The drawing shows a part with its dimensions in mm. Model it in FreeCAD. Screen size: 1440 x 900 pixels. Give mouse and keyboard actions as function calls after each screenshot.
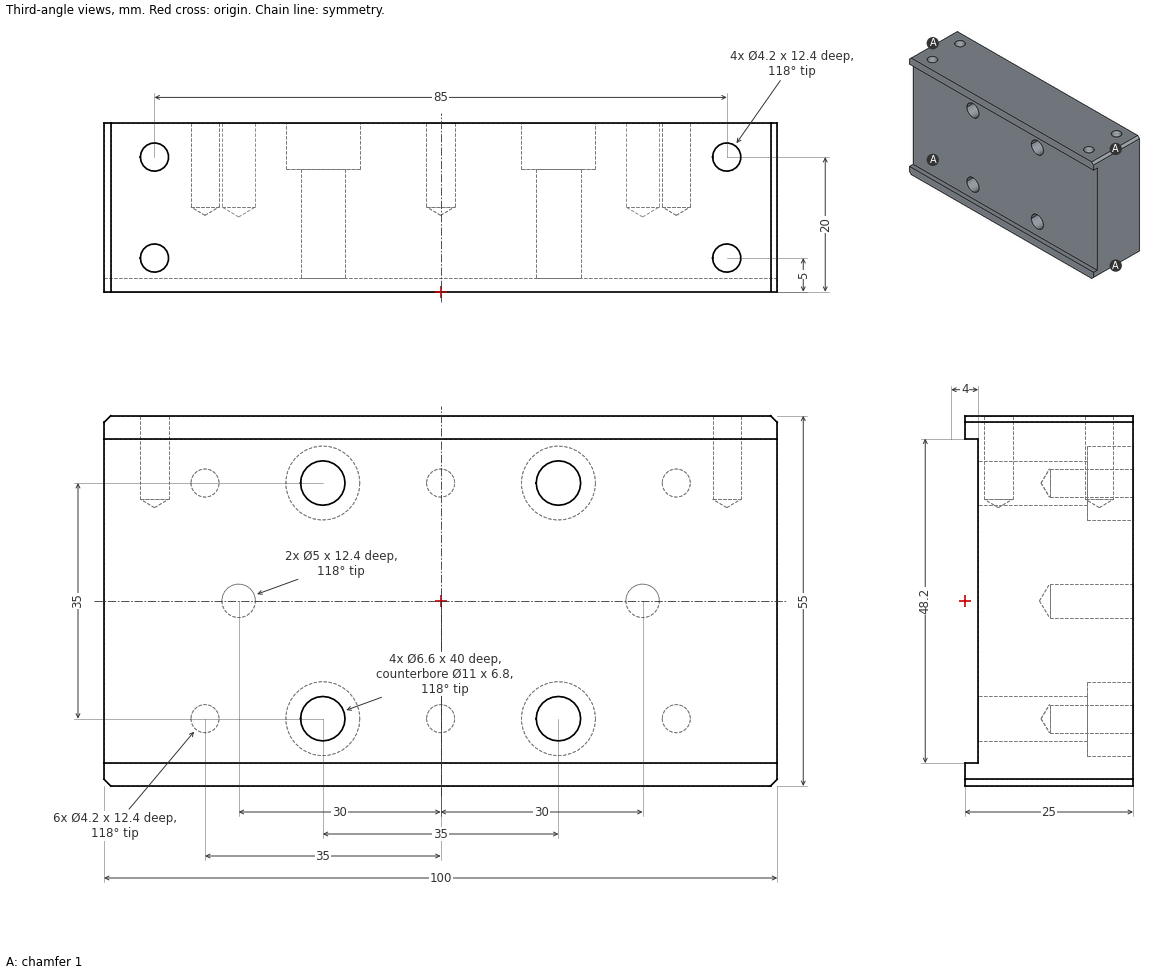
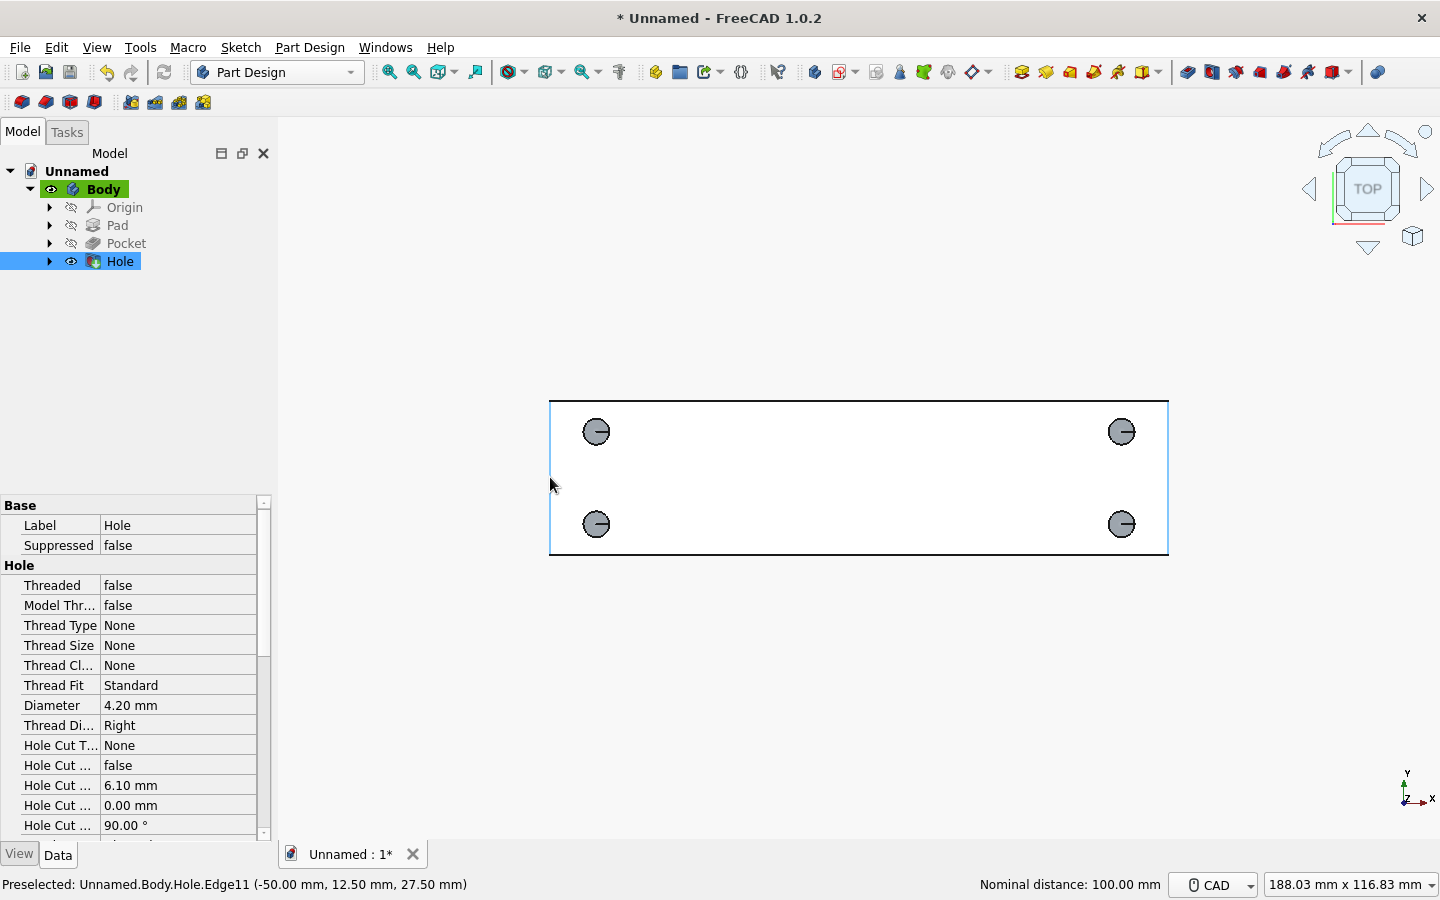
key(1)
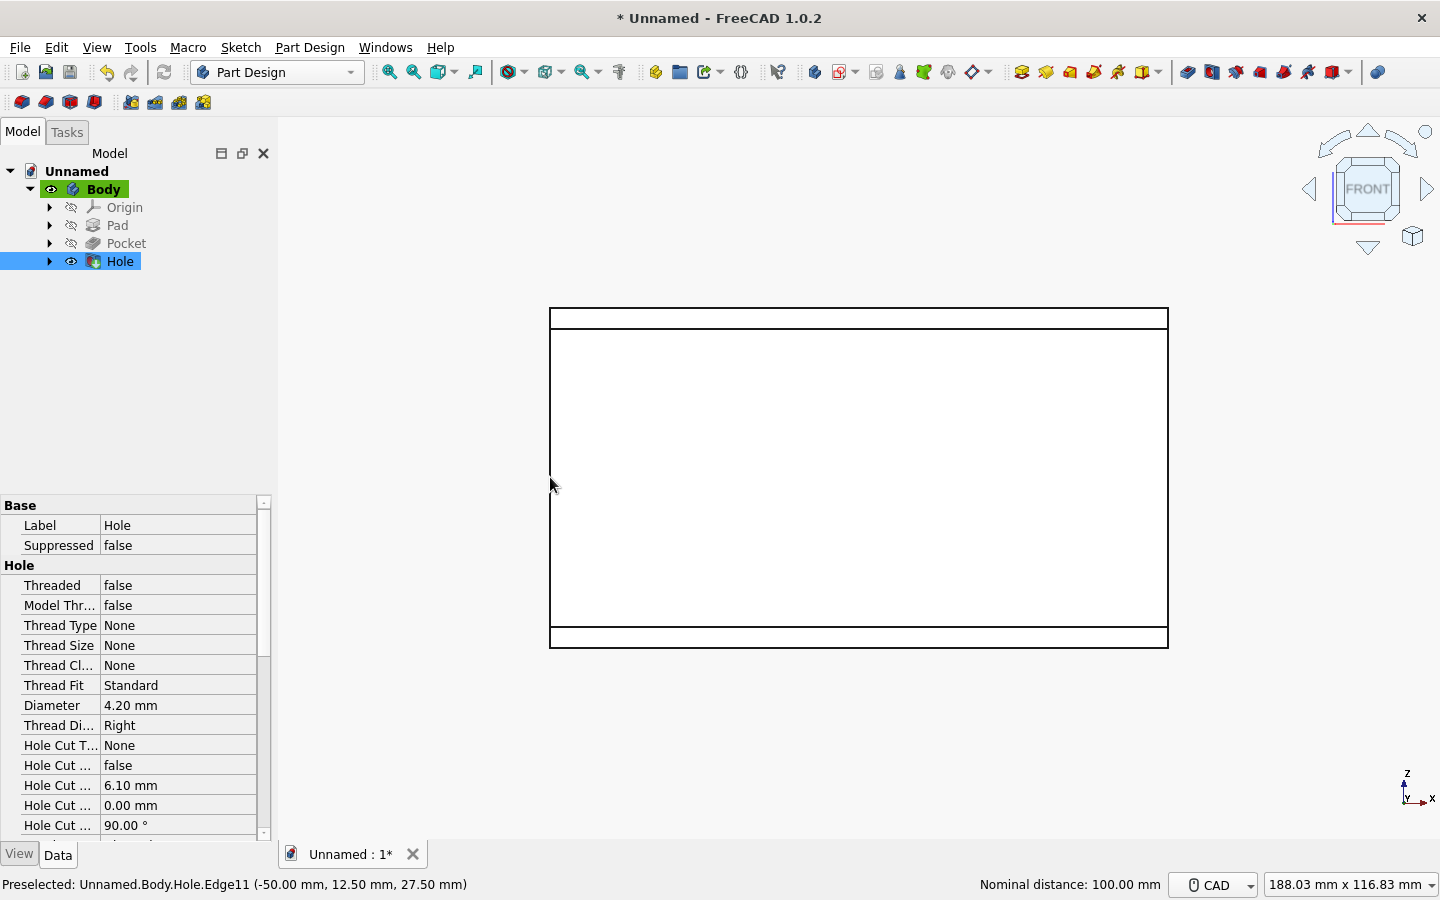
key(3)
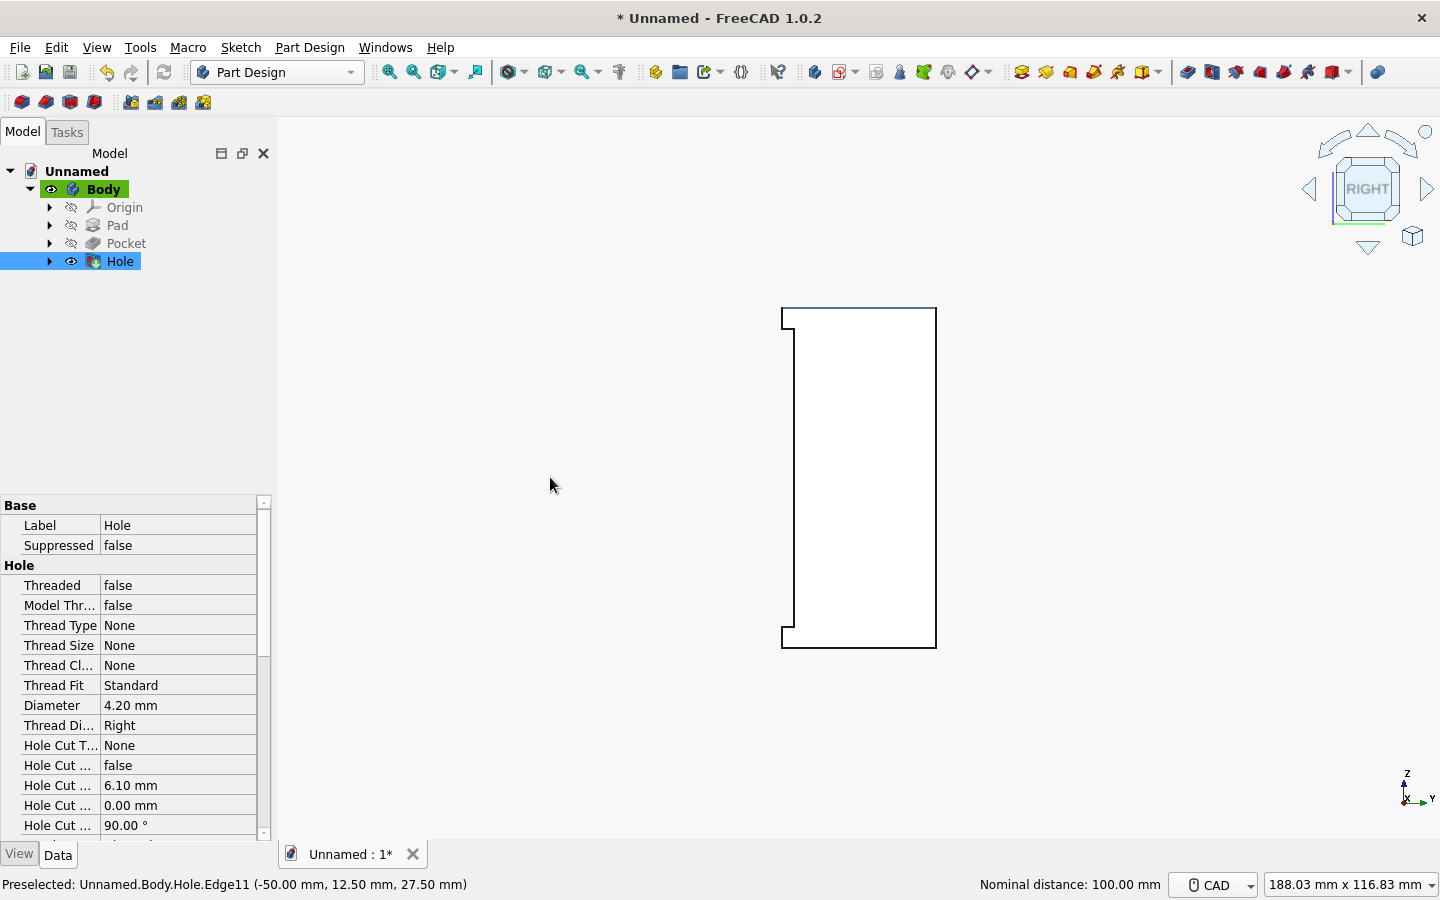
click(859, 647, ctrl)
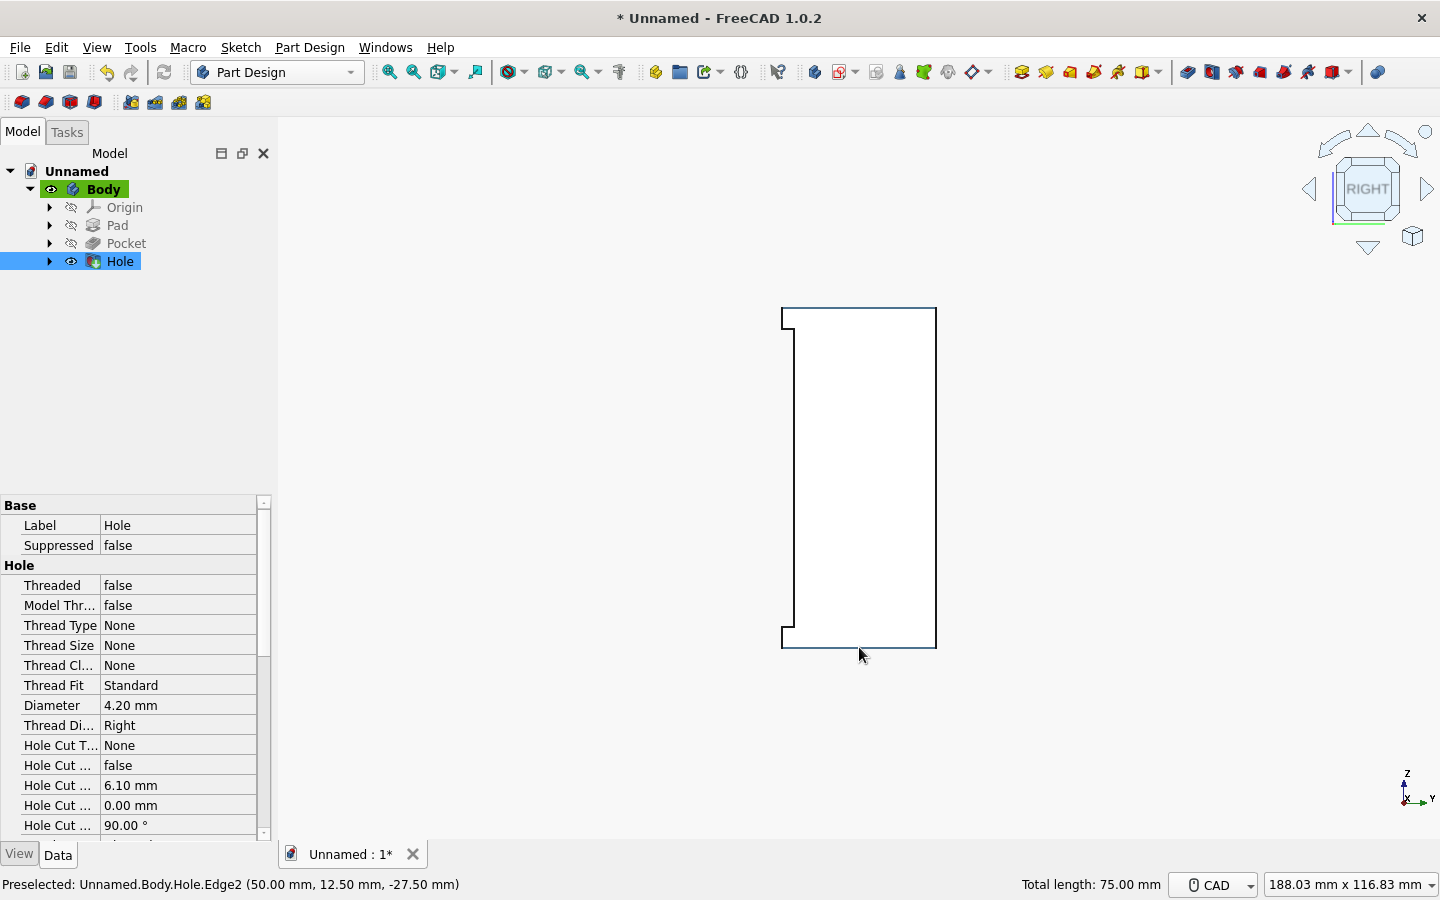
key(5)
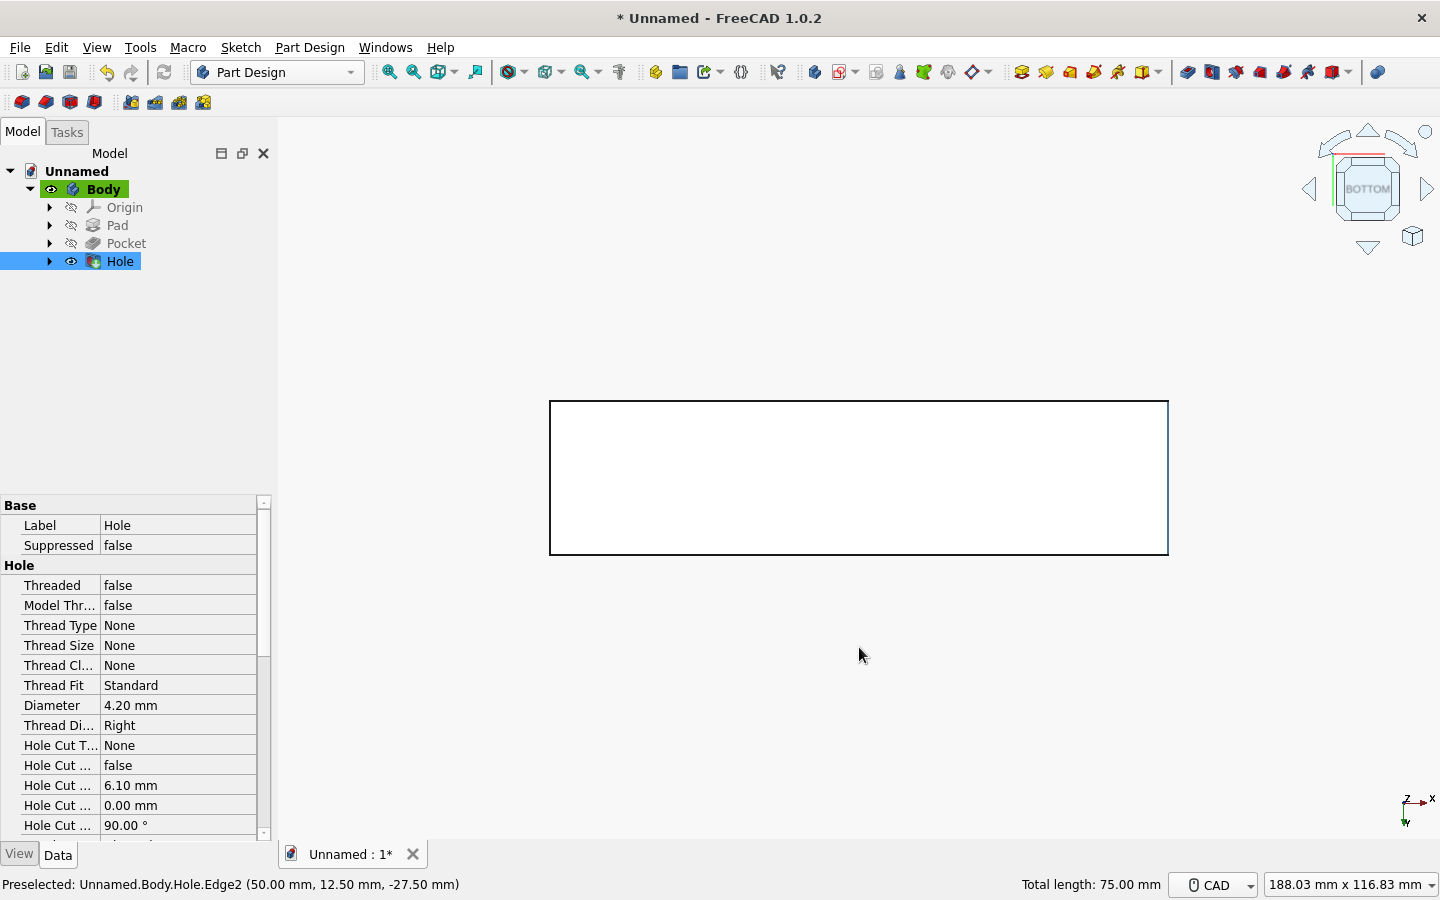
click(550, 477, ctrl)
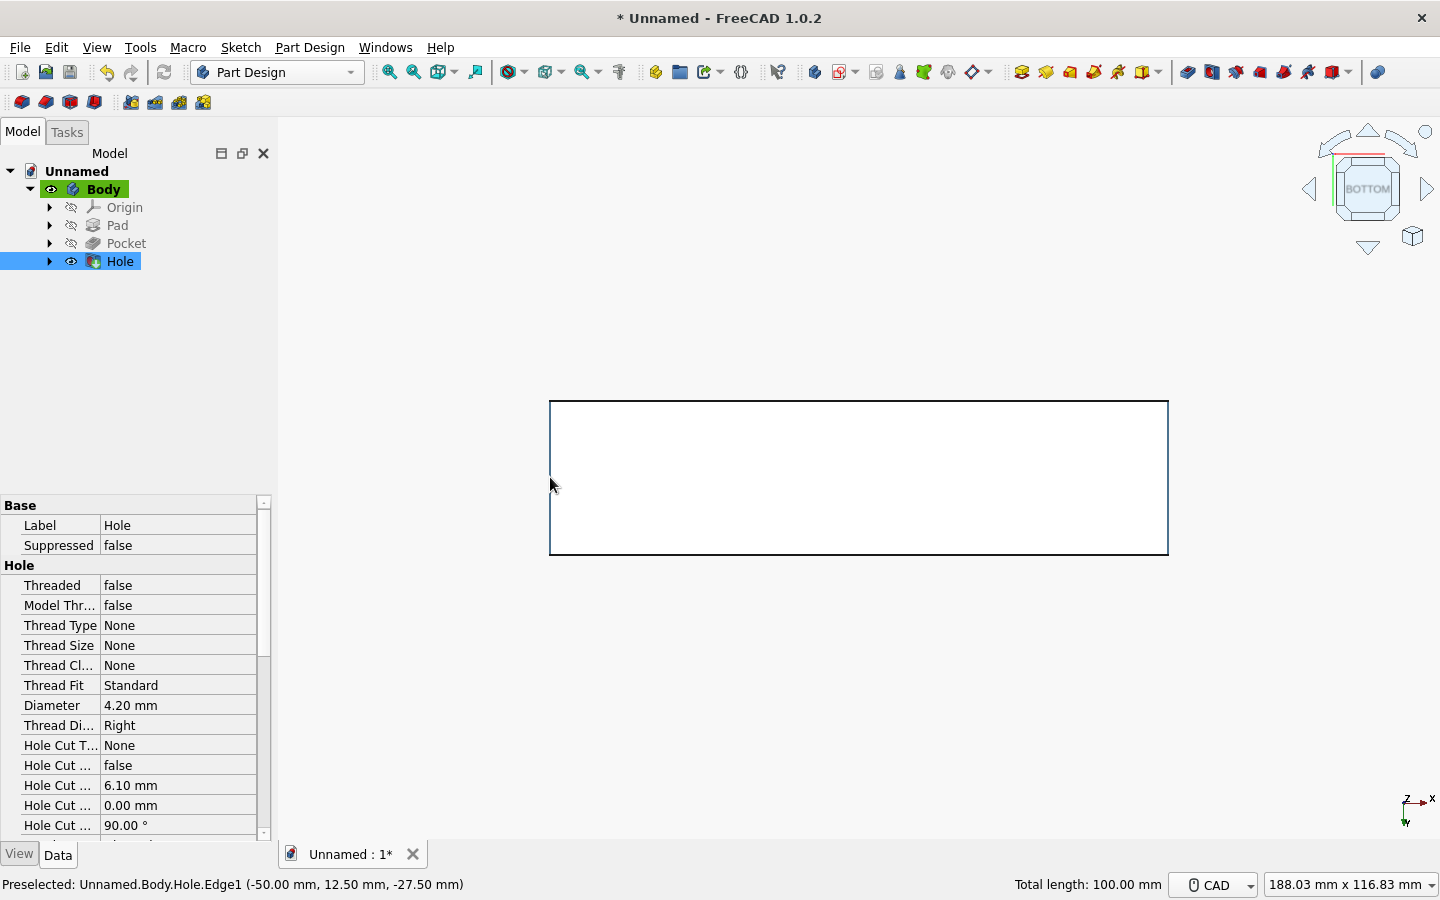
click(46, 102)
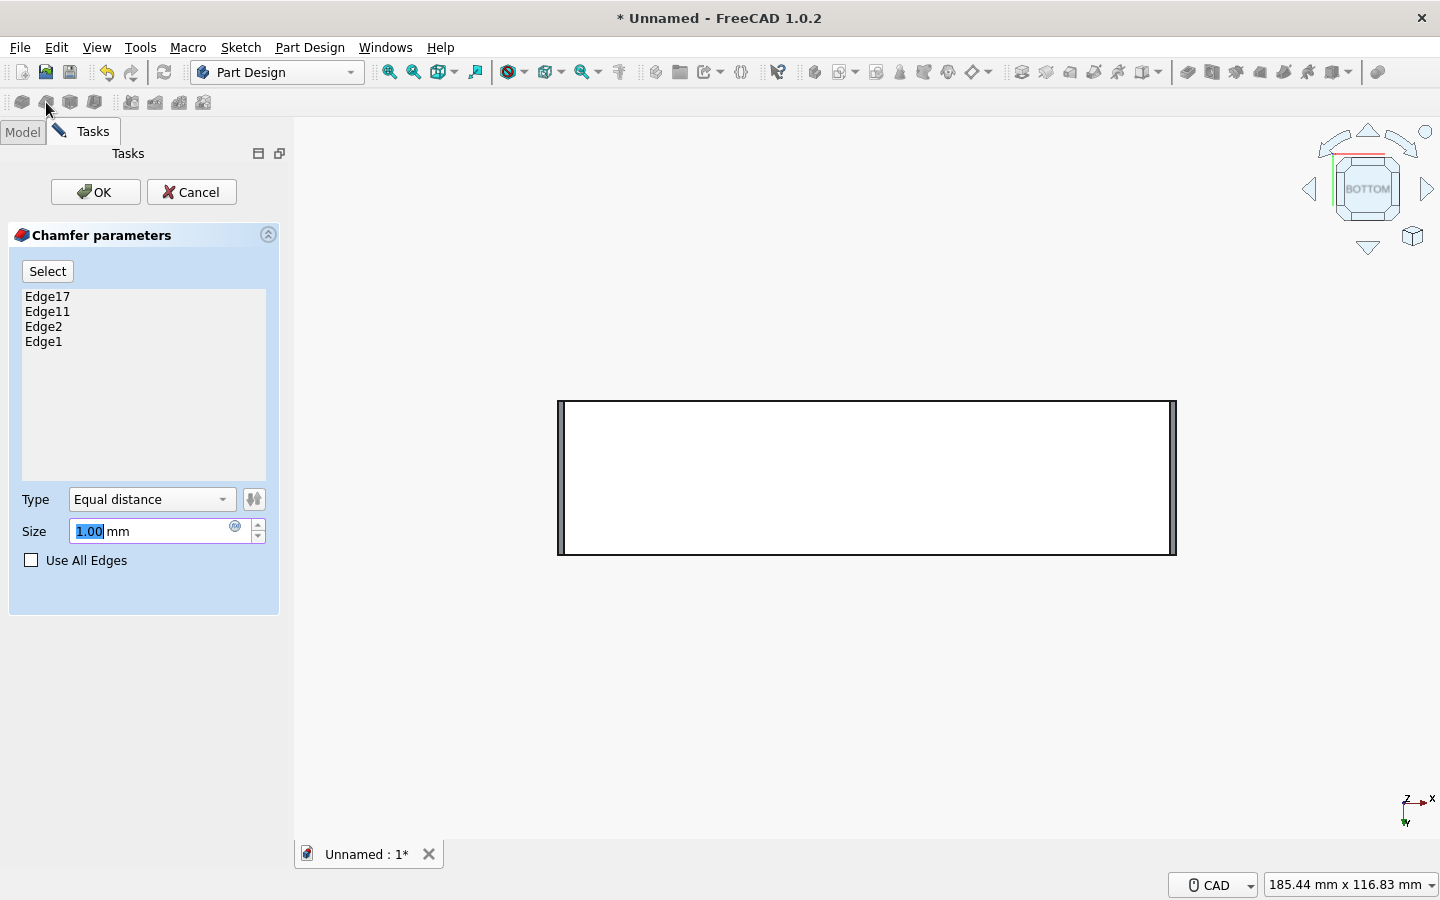
text(1)
key(Tab)